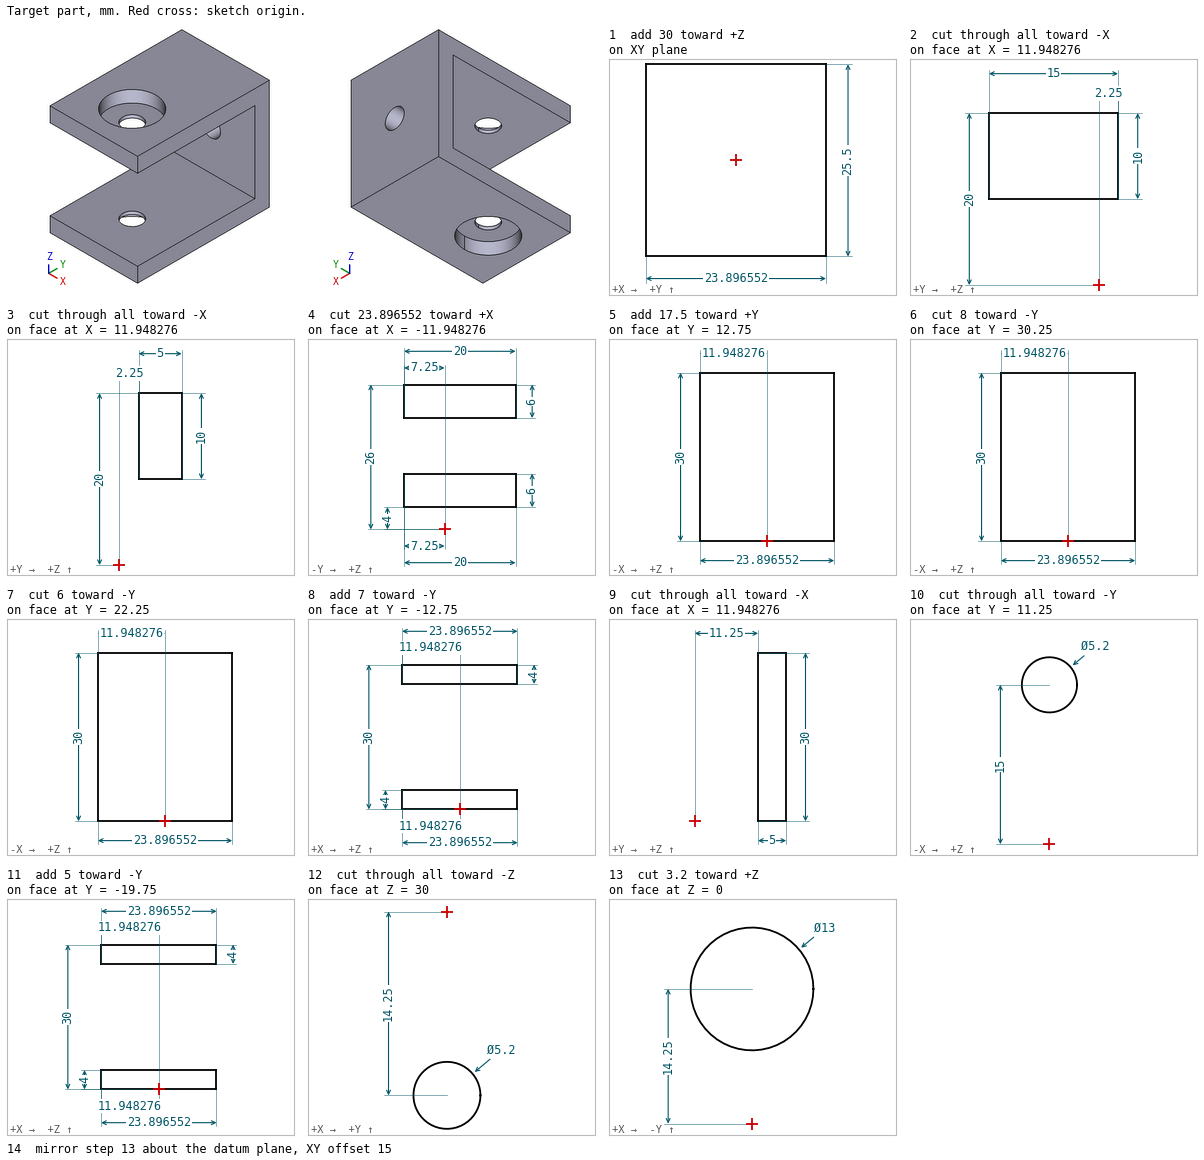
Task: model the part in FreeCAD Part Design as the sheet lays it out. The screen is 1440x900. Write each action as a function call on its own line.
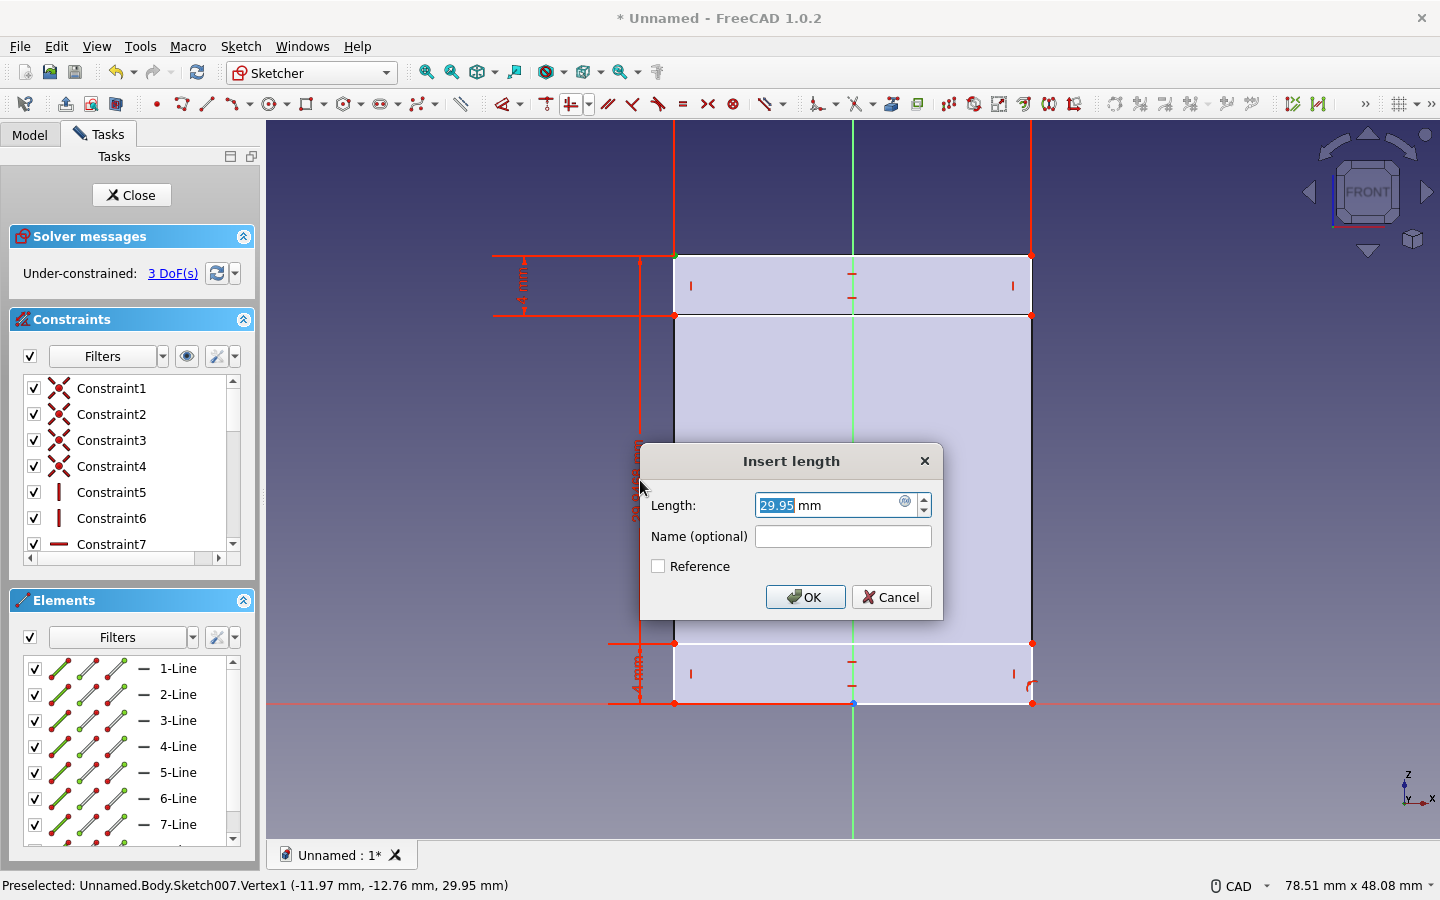
text(30)
key(Return)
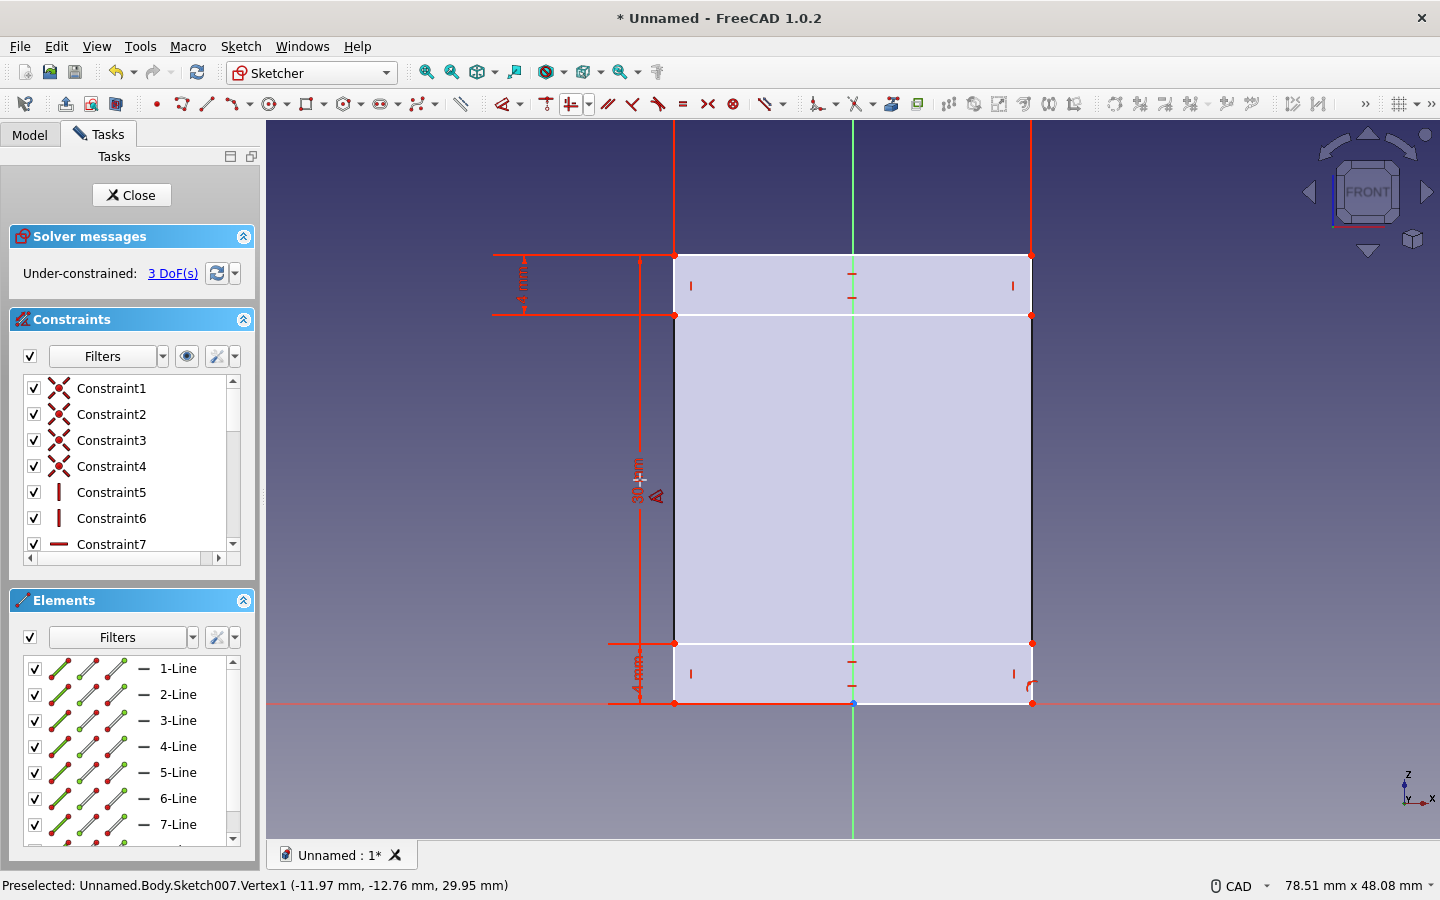
click(781, 704)
click(771, 738)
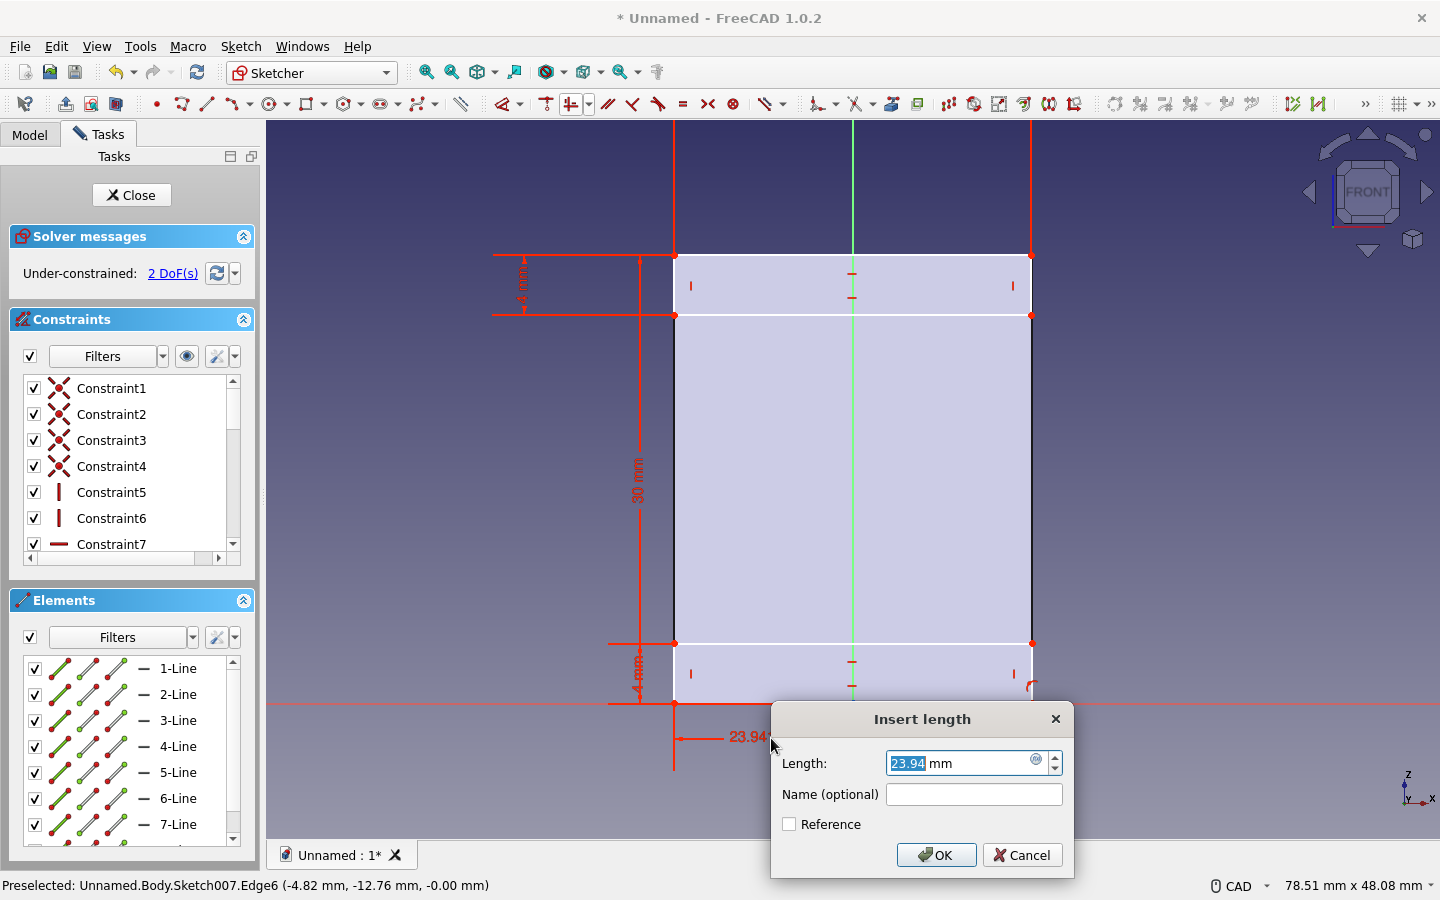
text(23.896552)
key(Return)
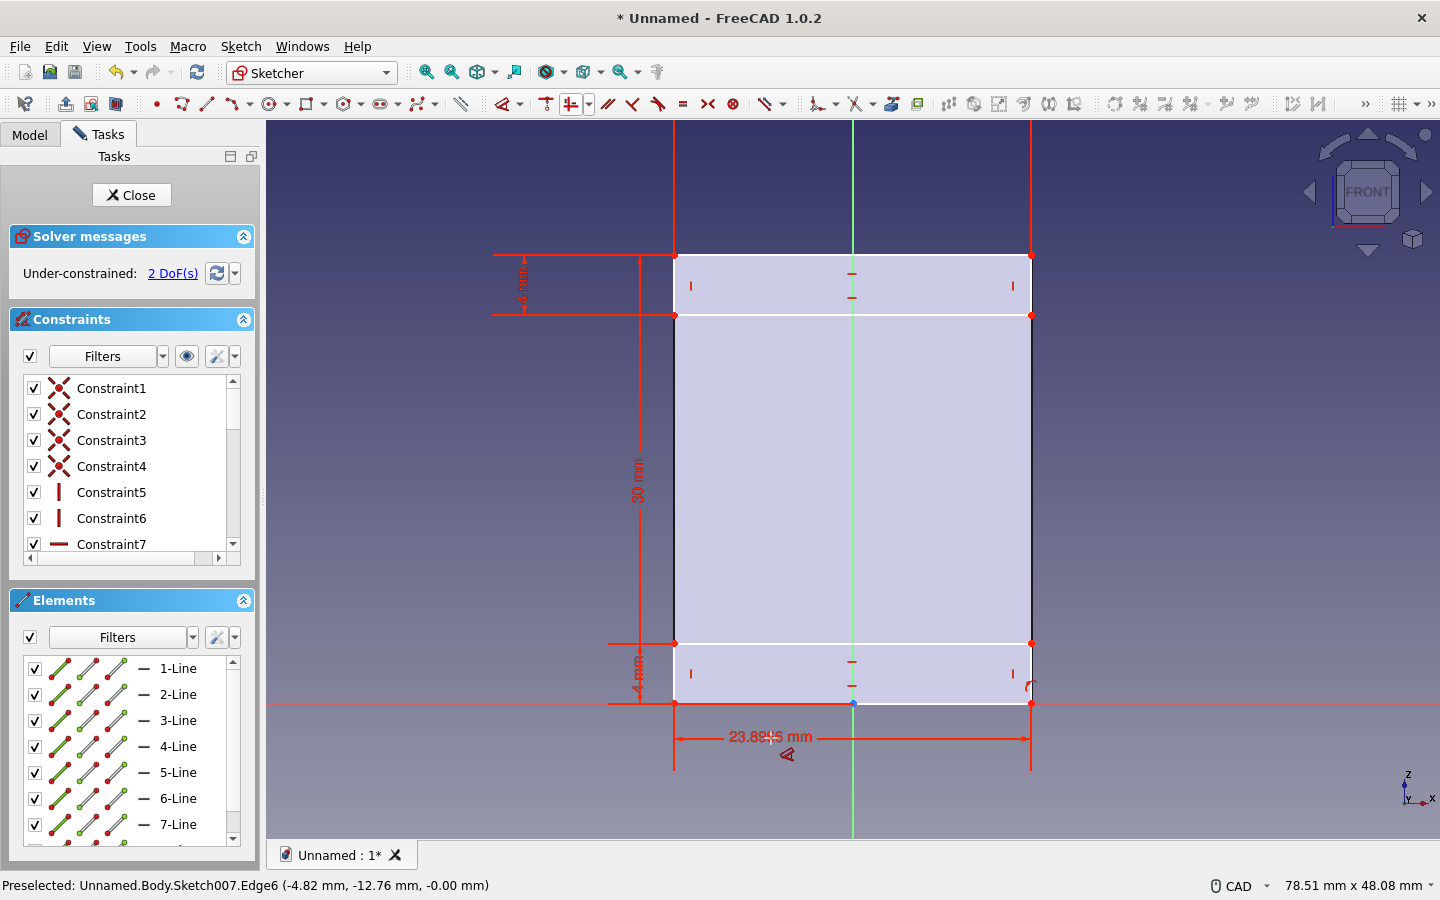
click(674, 255)
click(763, 221)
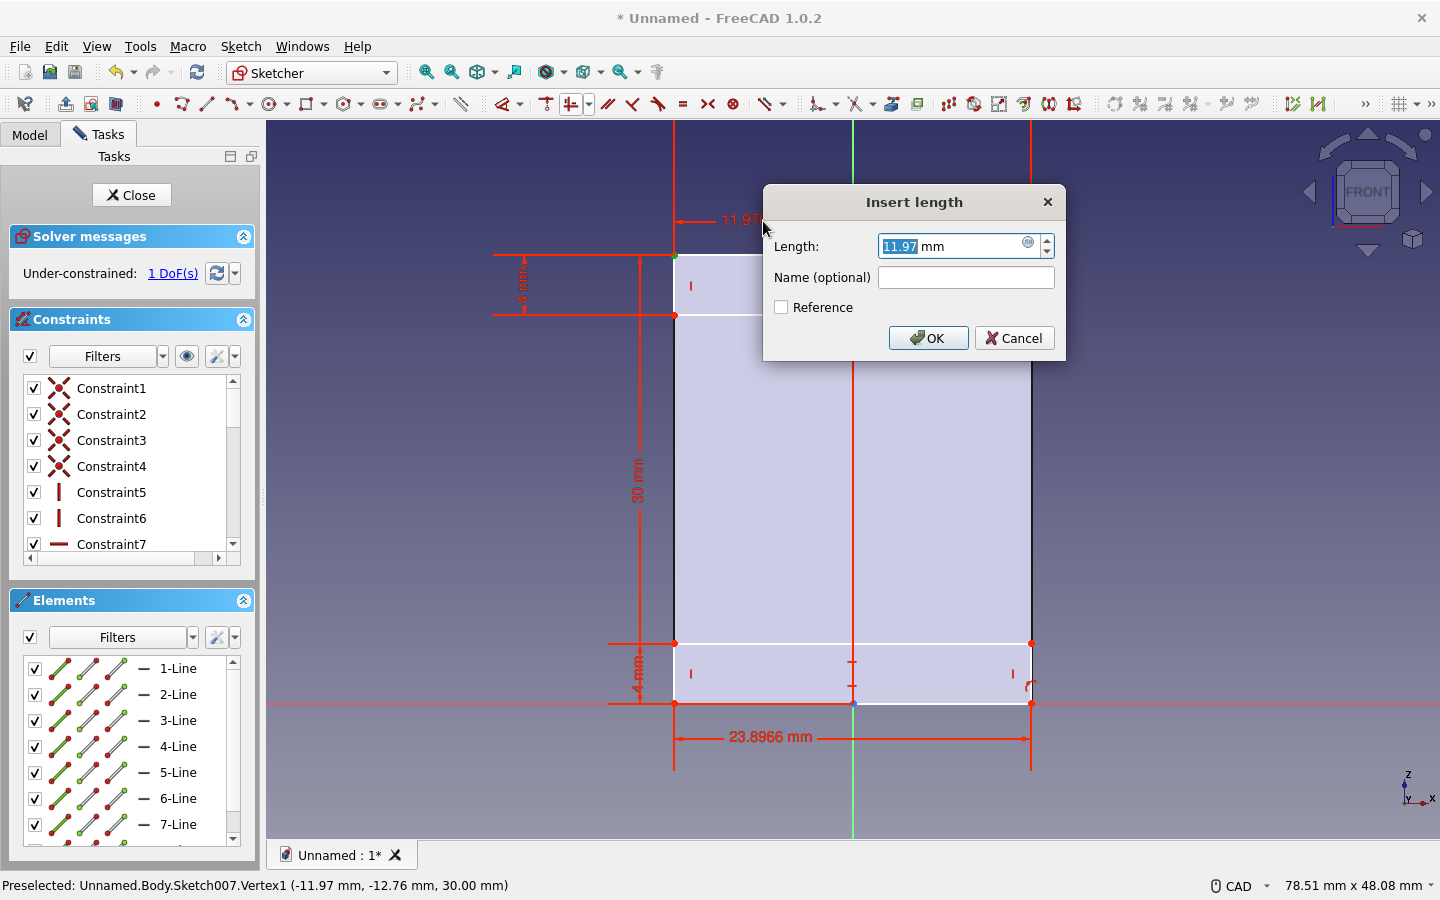
text(11.948276)
key(Return)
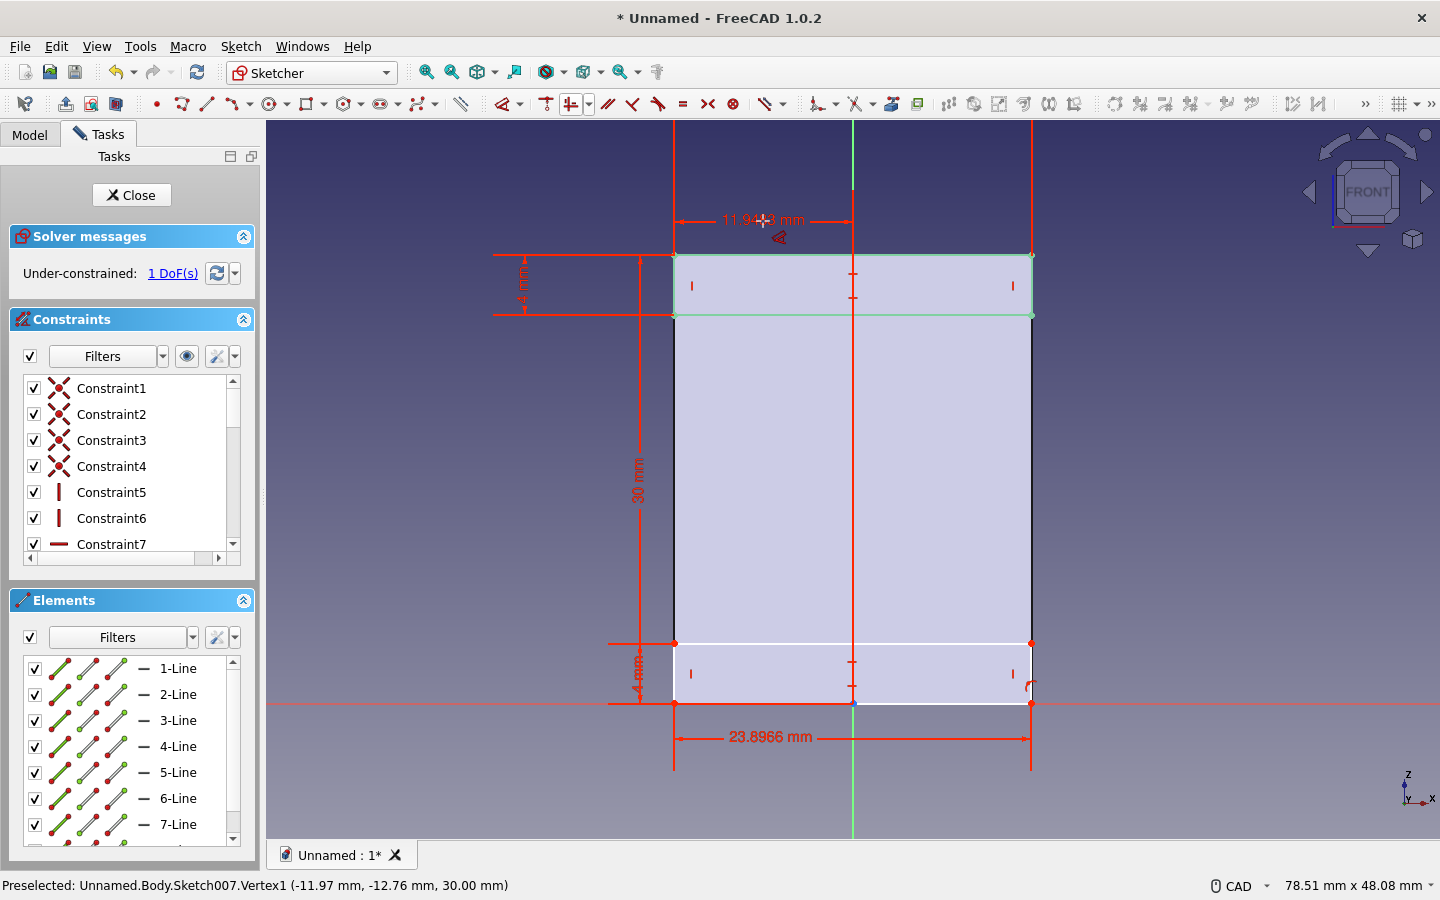
click(674, 644)
click(763, 610)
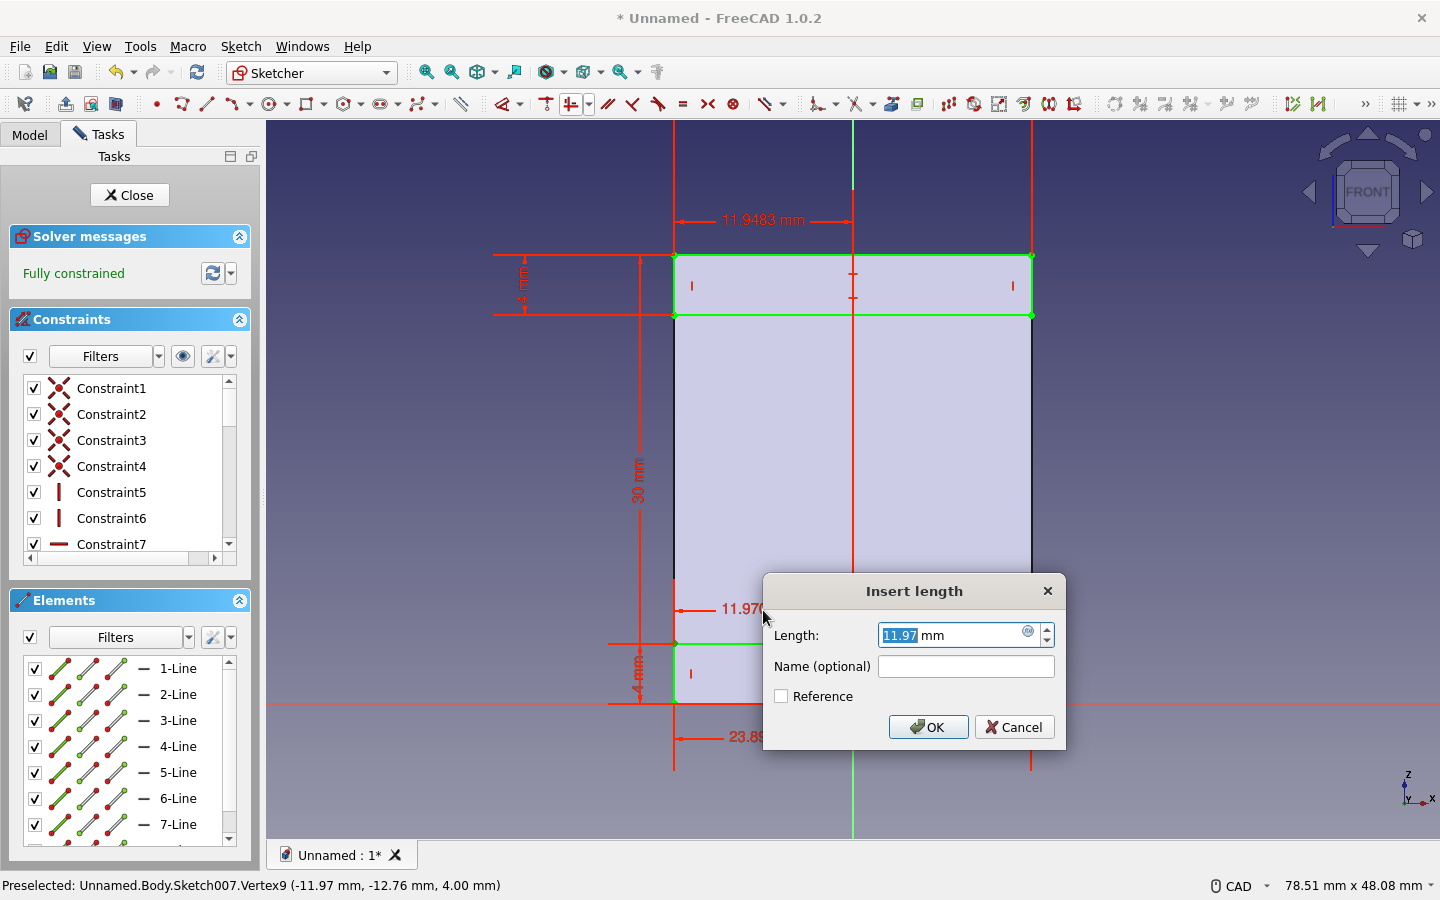
text(11.948276)
key(Return)
key(Escape)